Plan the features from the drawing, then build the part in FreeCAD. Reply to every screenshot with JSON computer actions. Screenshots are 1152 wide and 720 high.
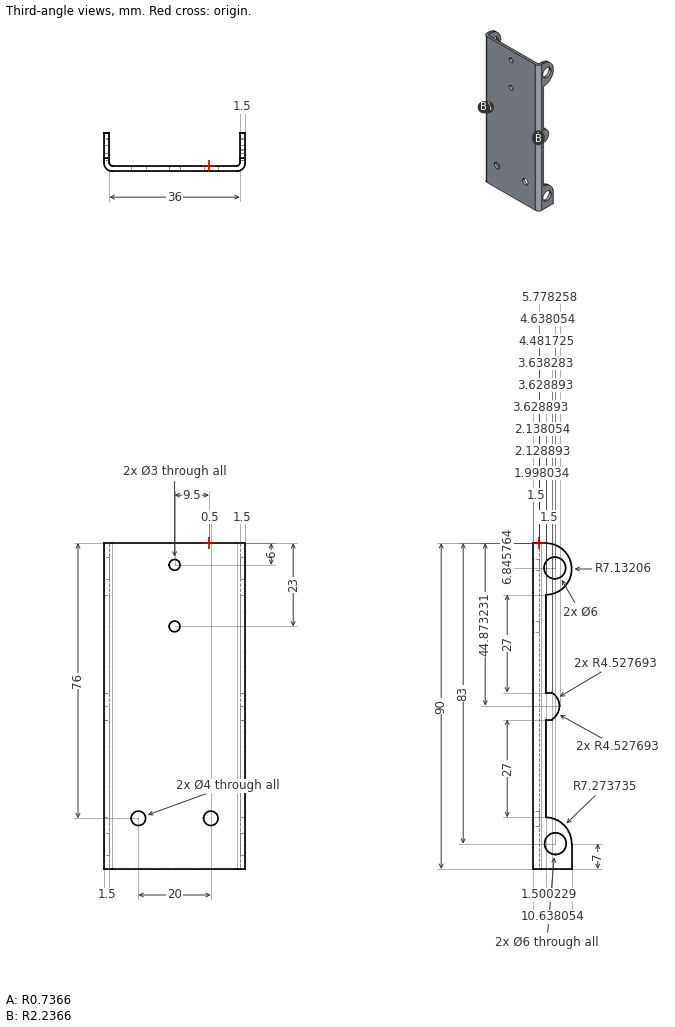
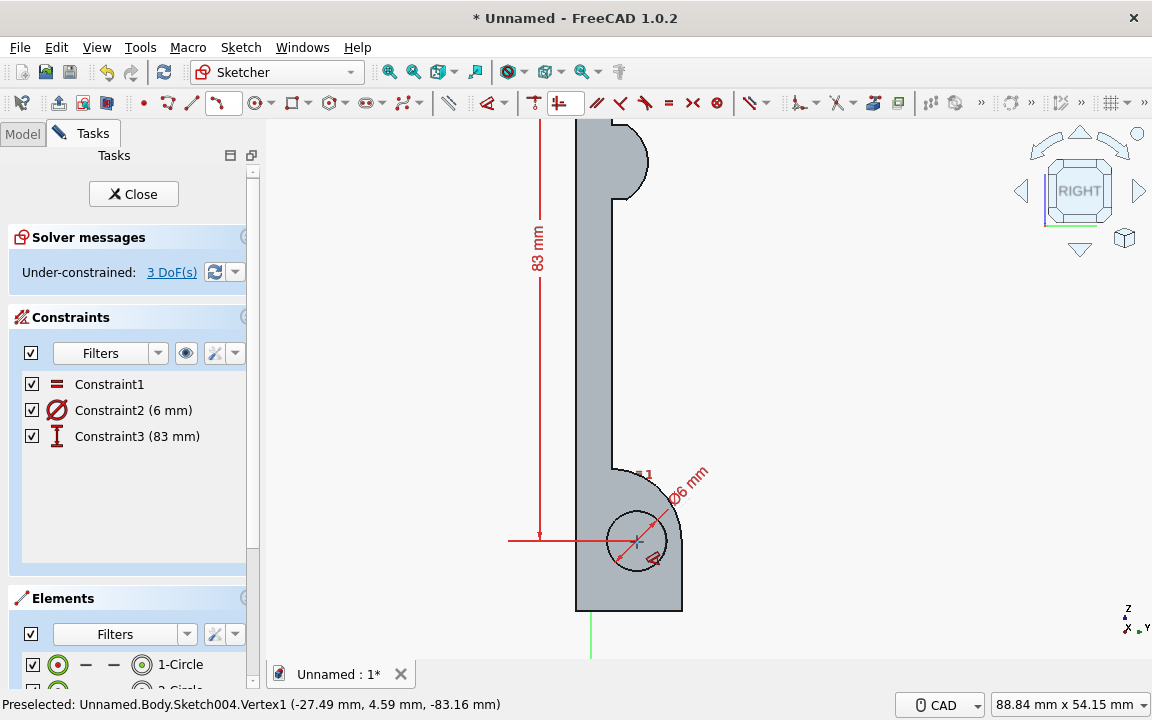
{"action": "left_click", "coordinate": [636, 541]}
{"action": "left_click", "coordinate": [613, 599]}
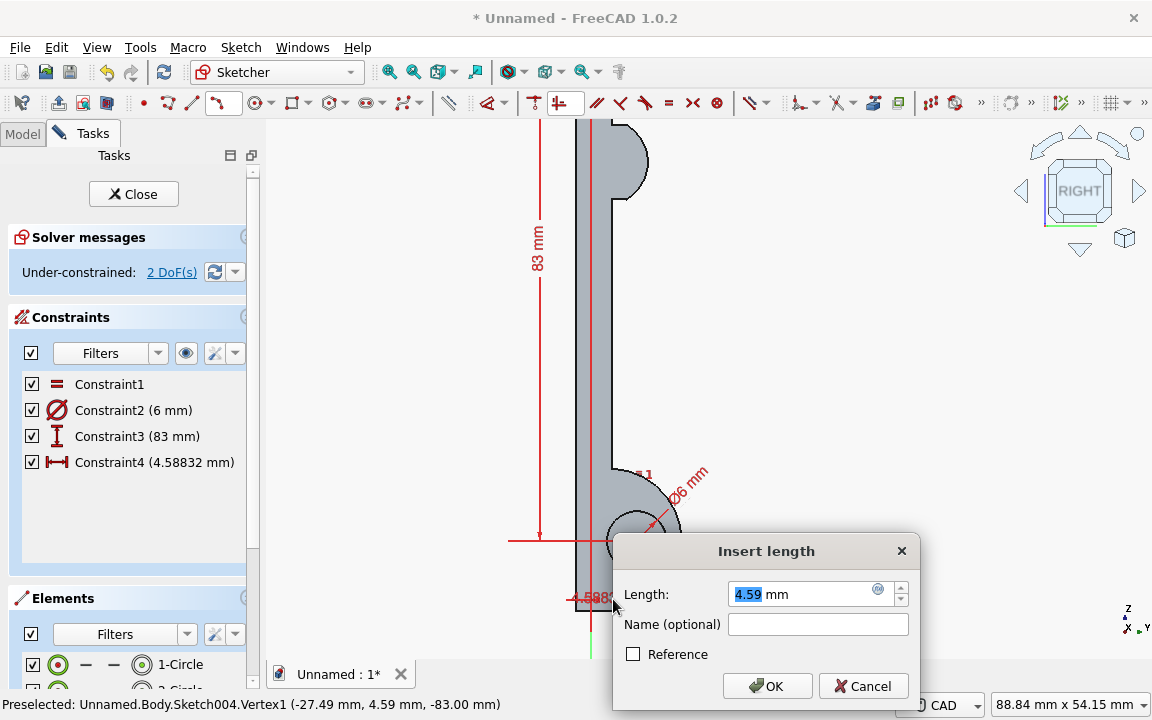
{"action": "type", "text": "4.638054"}
{"action": "key", "text": "Return"}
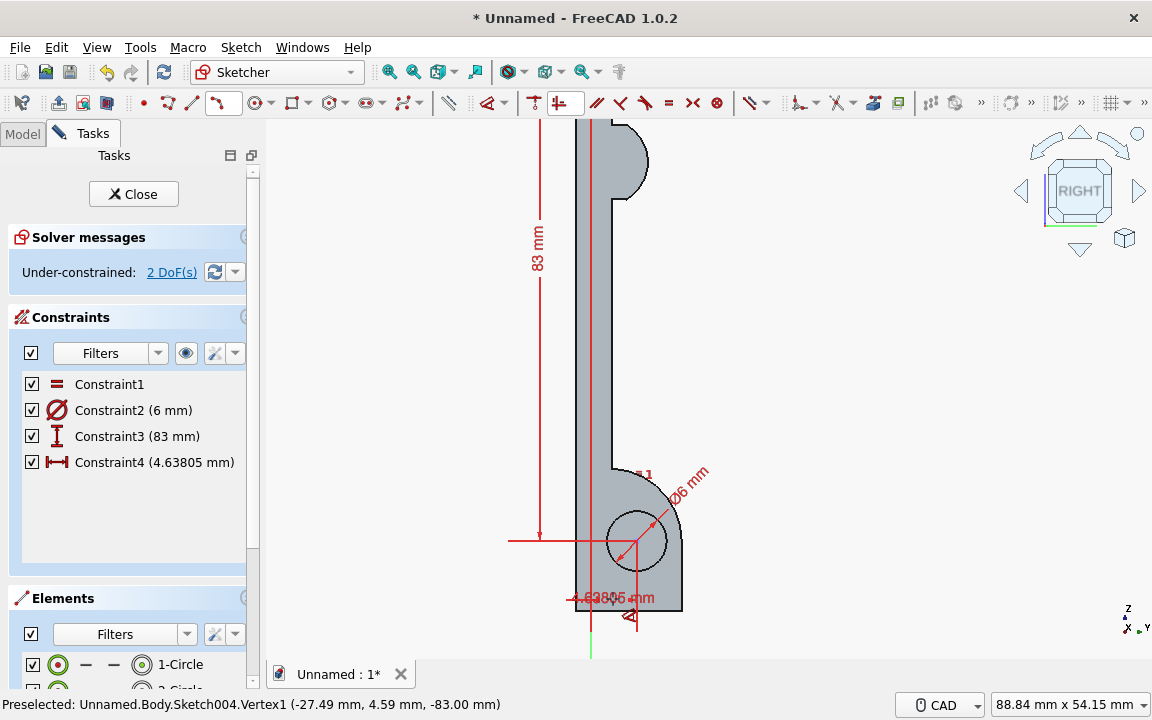
{"action": "scroll", "coordinate": [647, 533], "scroll_direction": "down", "scroll_amount": 5}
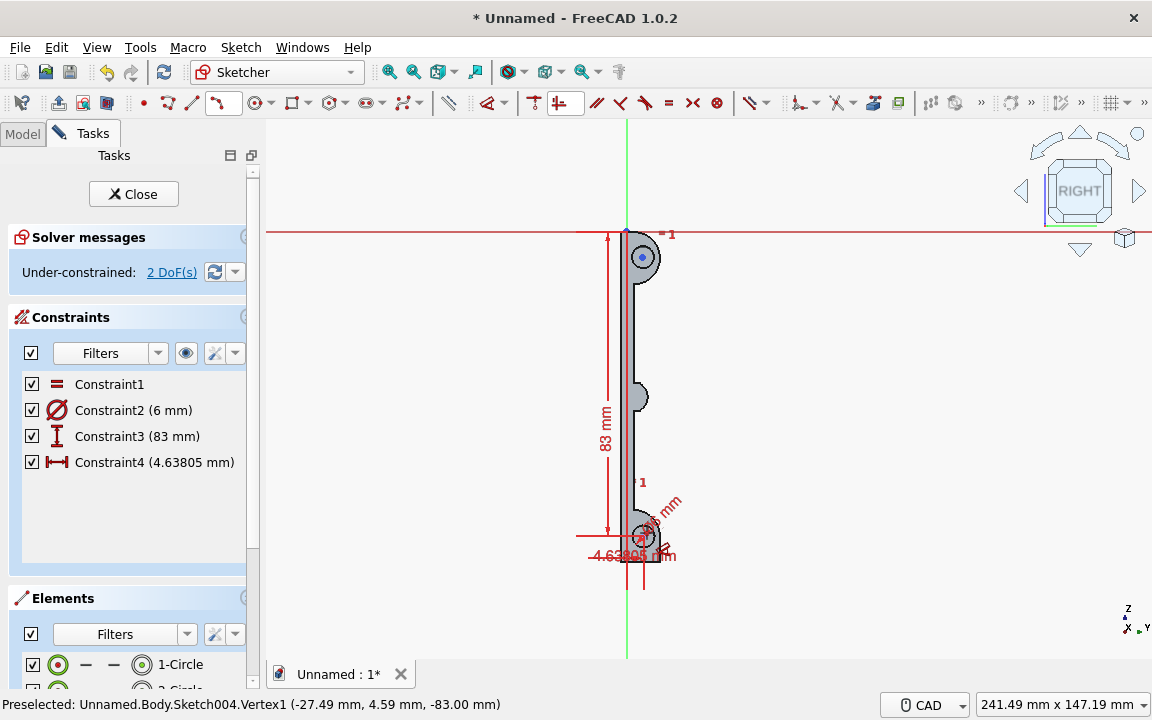
{"action": "scroll", "coordinate": [643, 258], "scroll_direction": "up", "scroll_amount": 5}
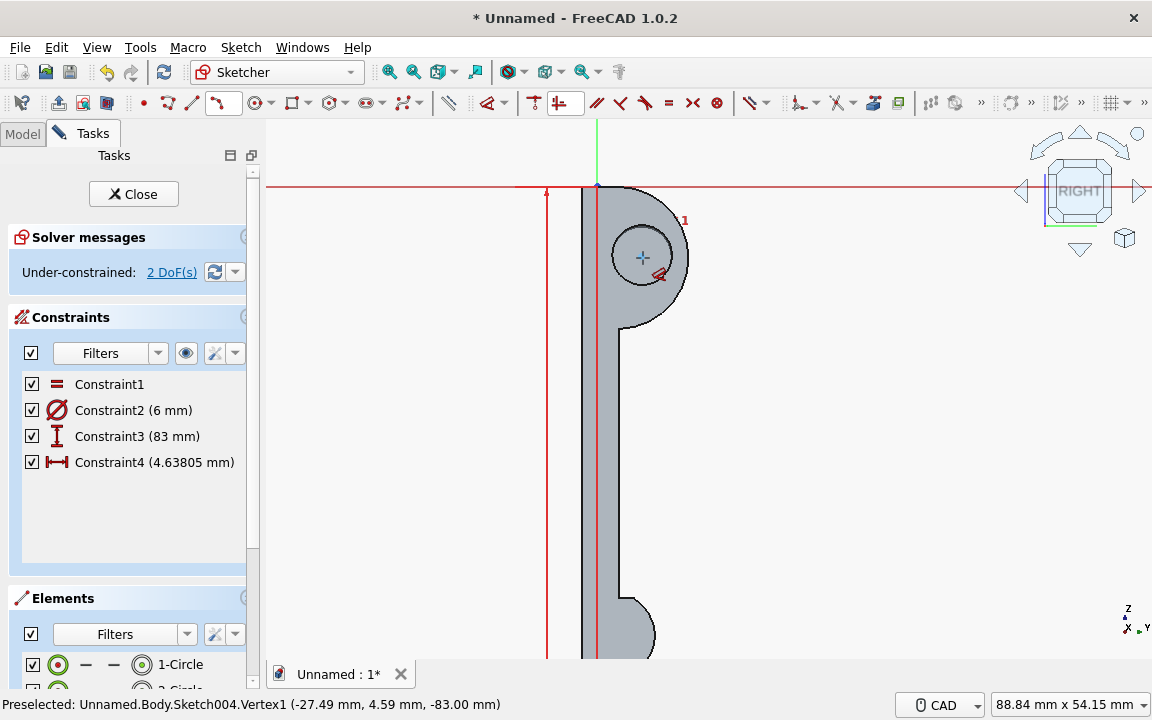
{"action": "left_click", "coordinate": [642, 257]}
{"action": "left_click", "coordinate": [620, 153]}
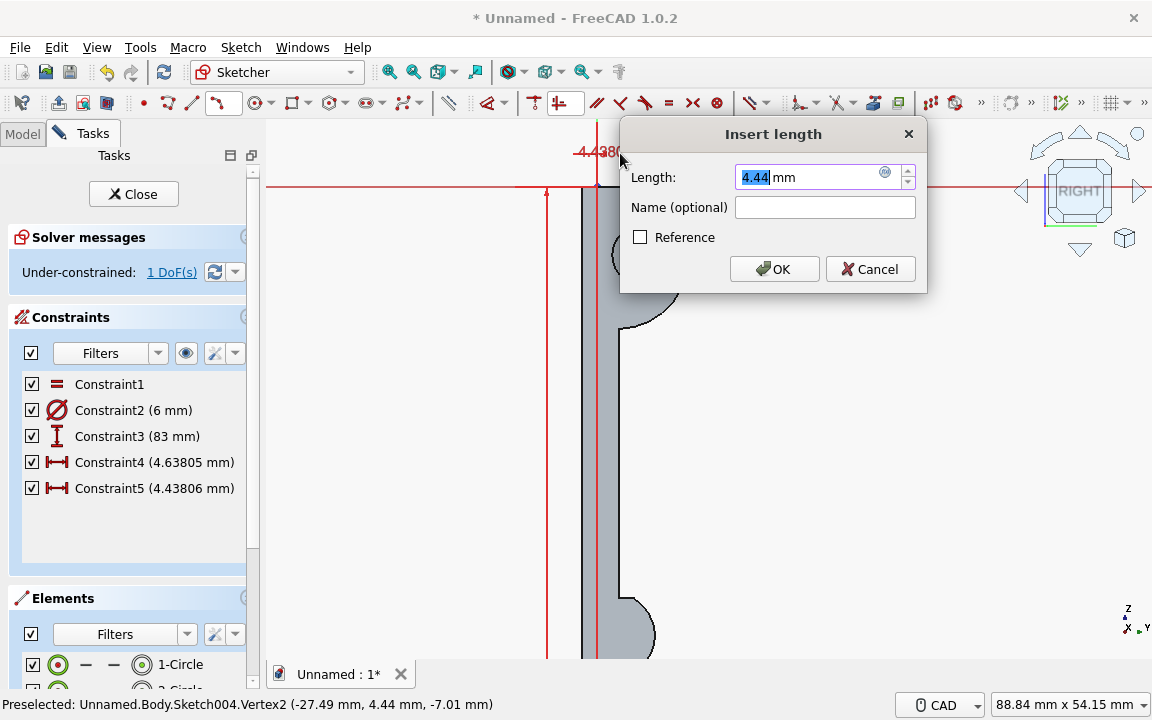
{"action": "type", "text": "4.481725"}
{"action": "key", "text": "Return"}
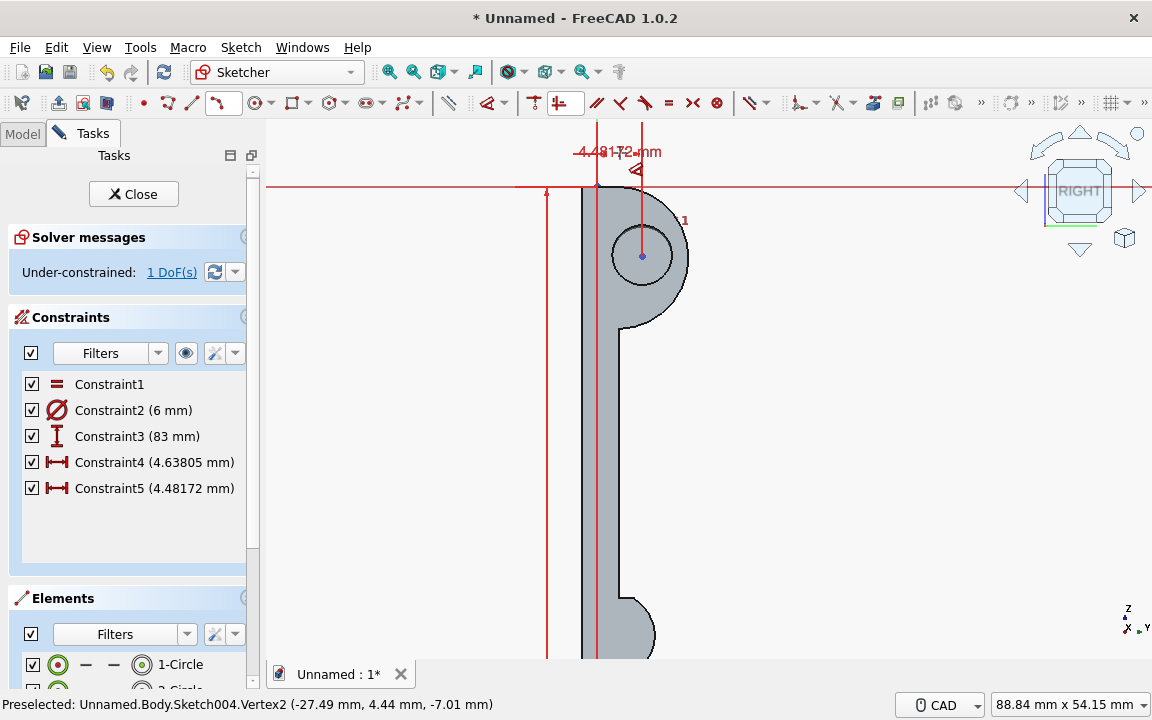
{"action": "left_click", "coordinate": [642, 257]}
{"action": "left_click", "coordinate": [563, 222]}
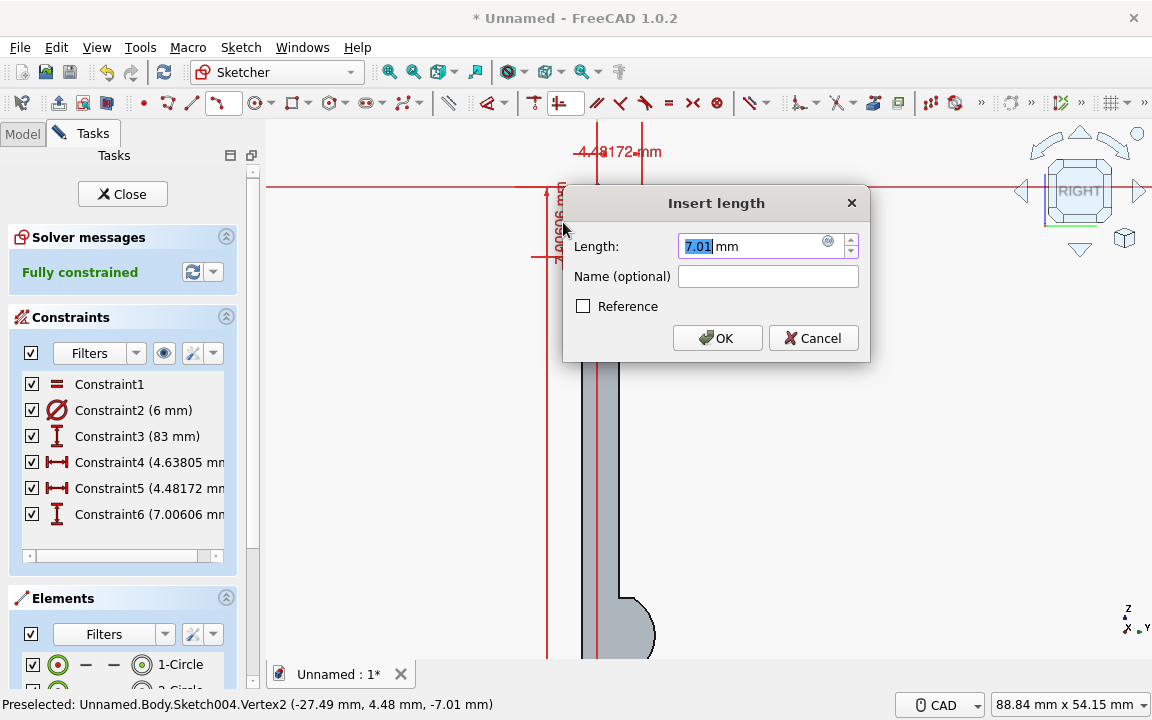
{"action": "type", "text": "6.845764"}
{"action": "key", "text": "Return"}
{"action": "key", "text": "Escape"}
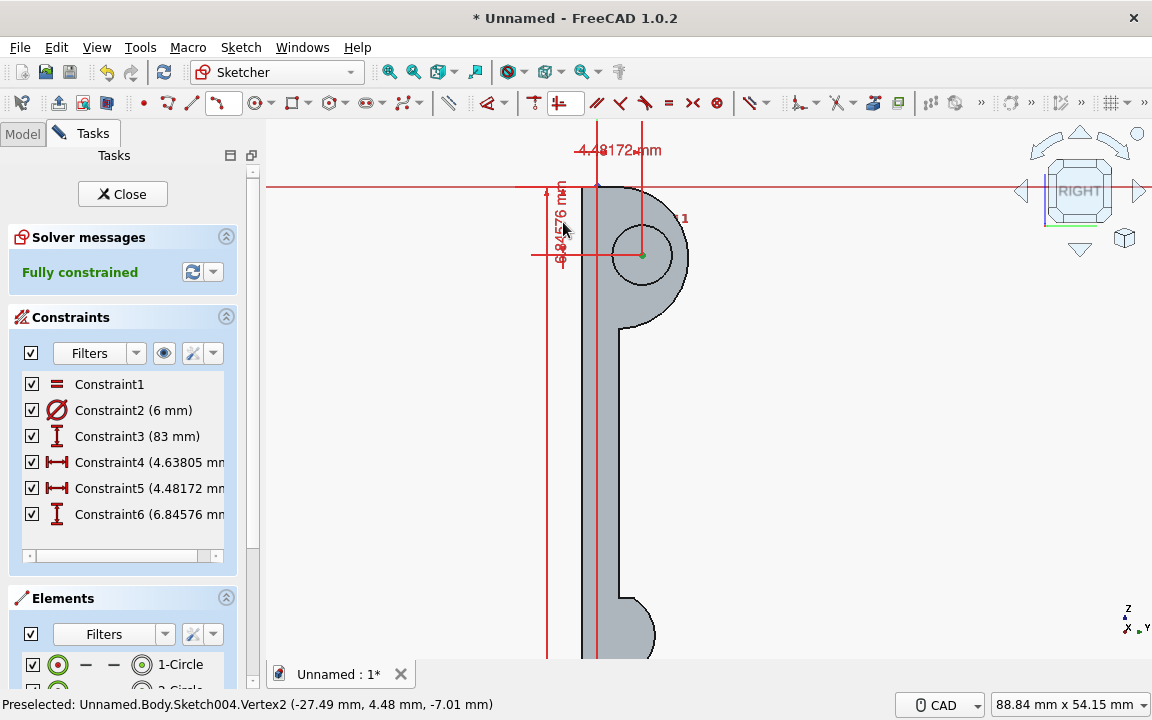
{"action": "left_click", "coordinate": [123, 194]}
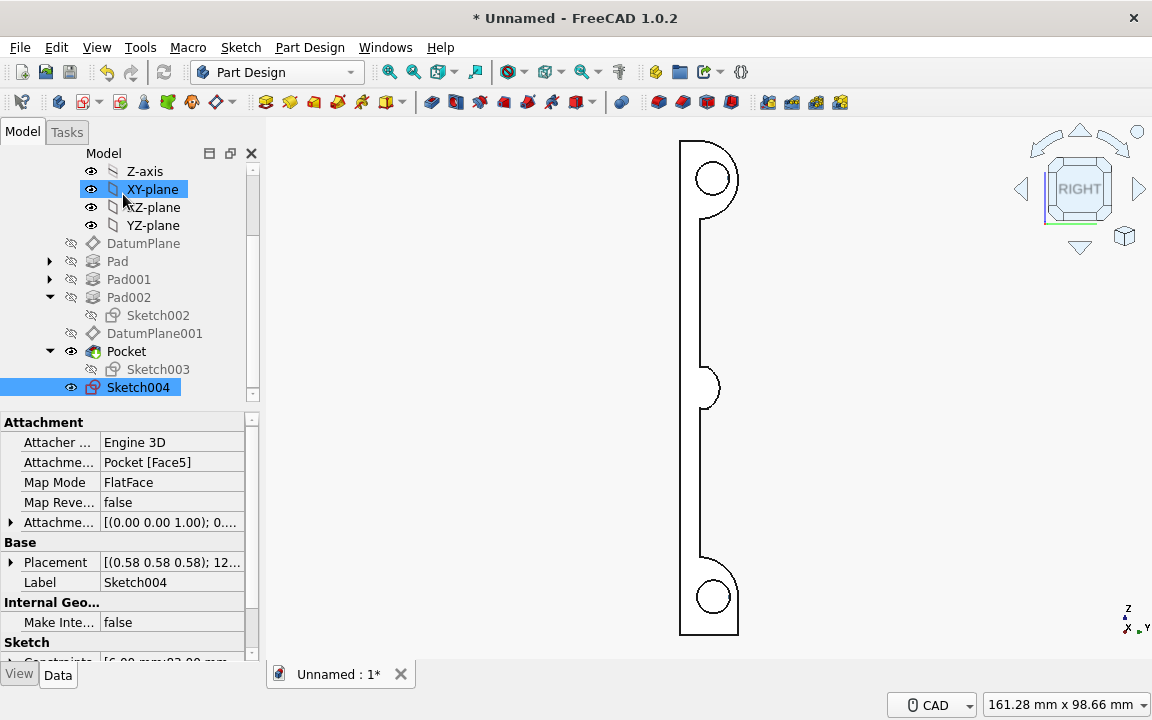
{"action": "left_click", "coordinate": [456, 102]}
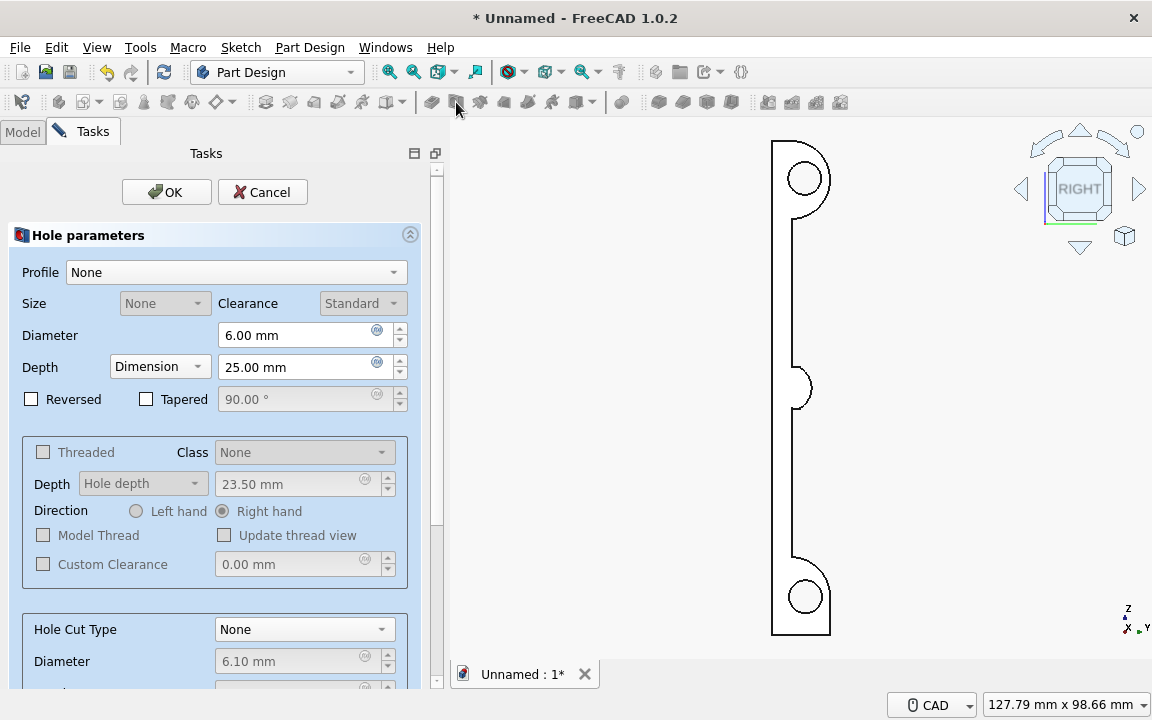
{"action": "triple_click", "coordinate": [305, 335]}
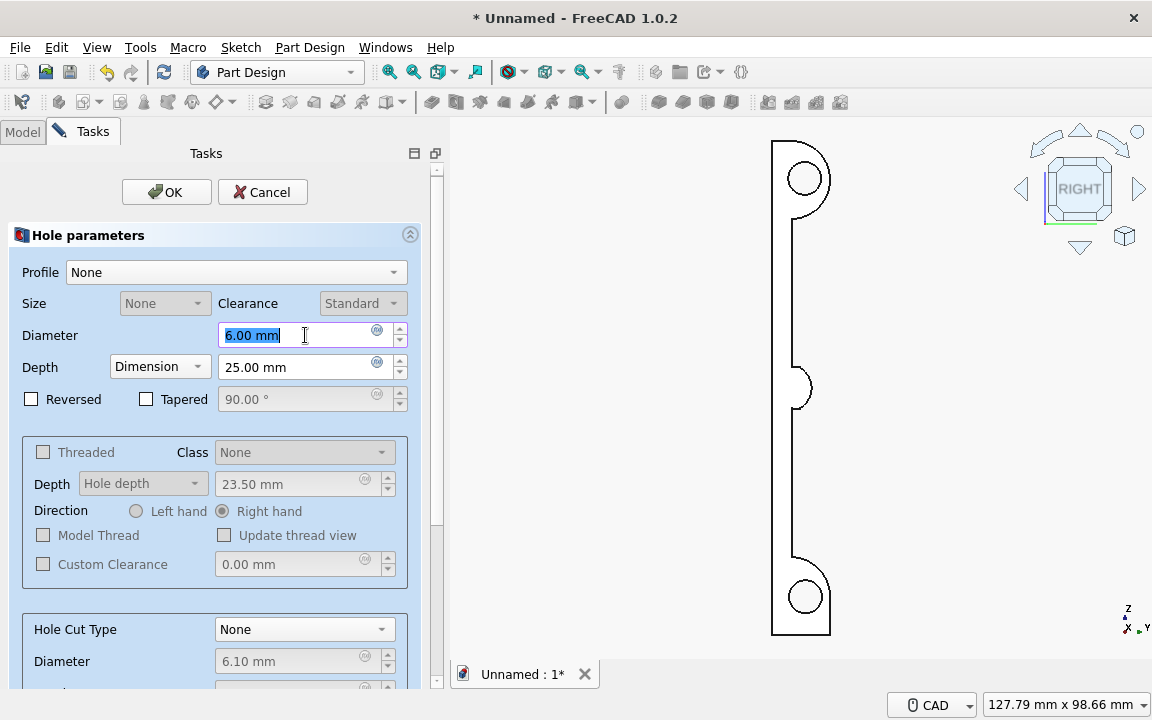
{"action": "type", "text": "6"}
{"action": "key", "text": "Tab"}